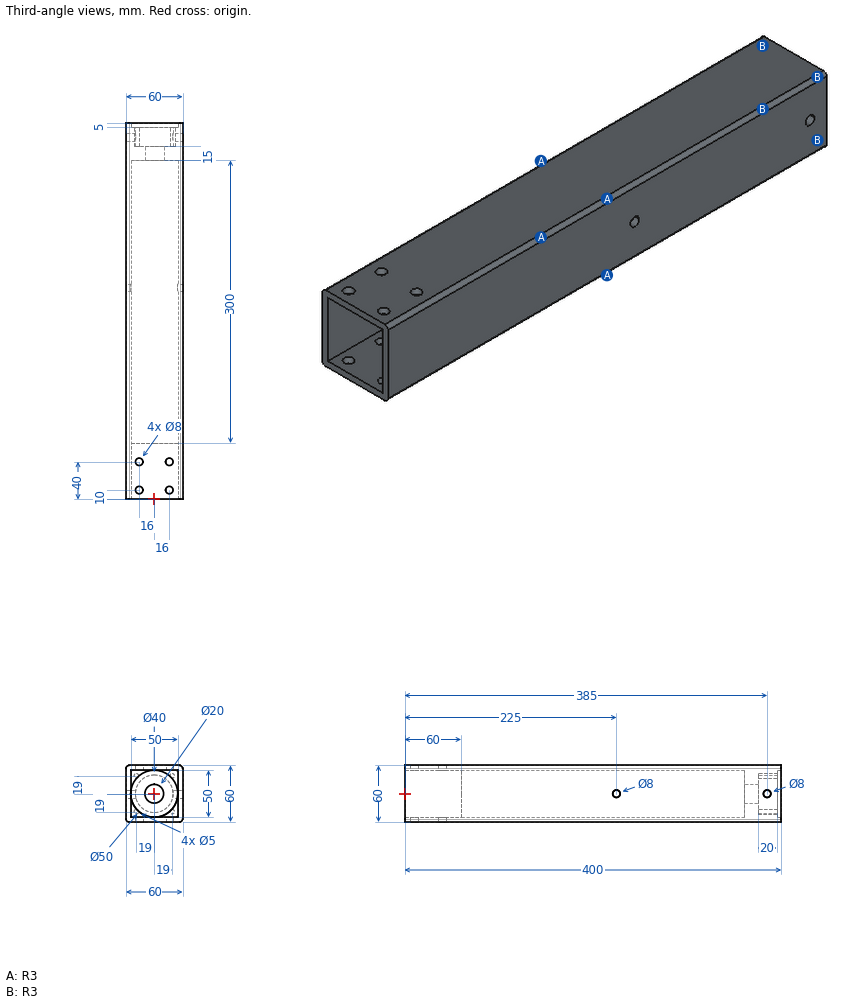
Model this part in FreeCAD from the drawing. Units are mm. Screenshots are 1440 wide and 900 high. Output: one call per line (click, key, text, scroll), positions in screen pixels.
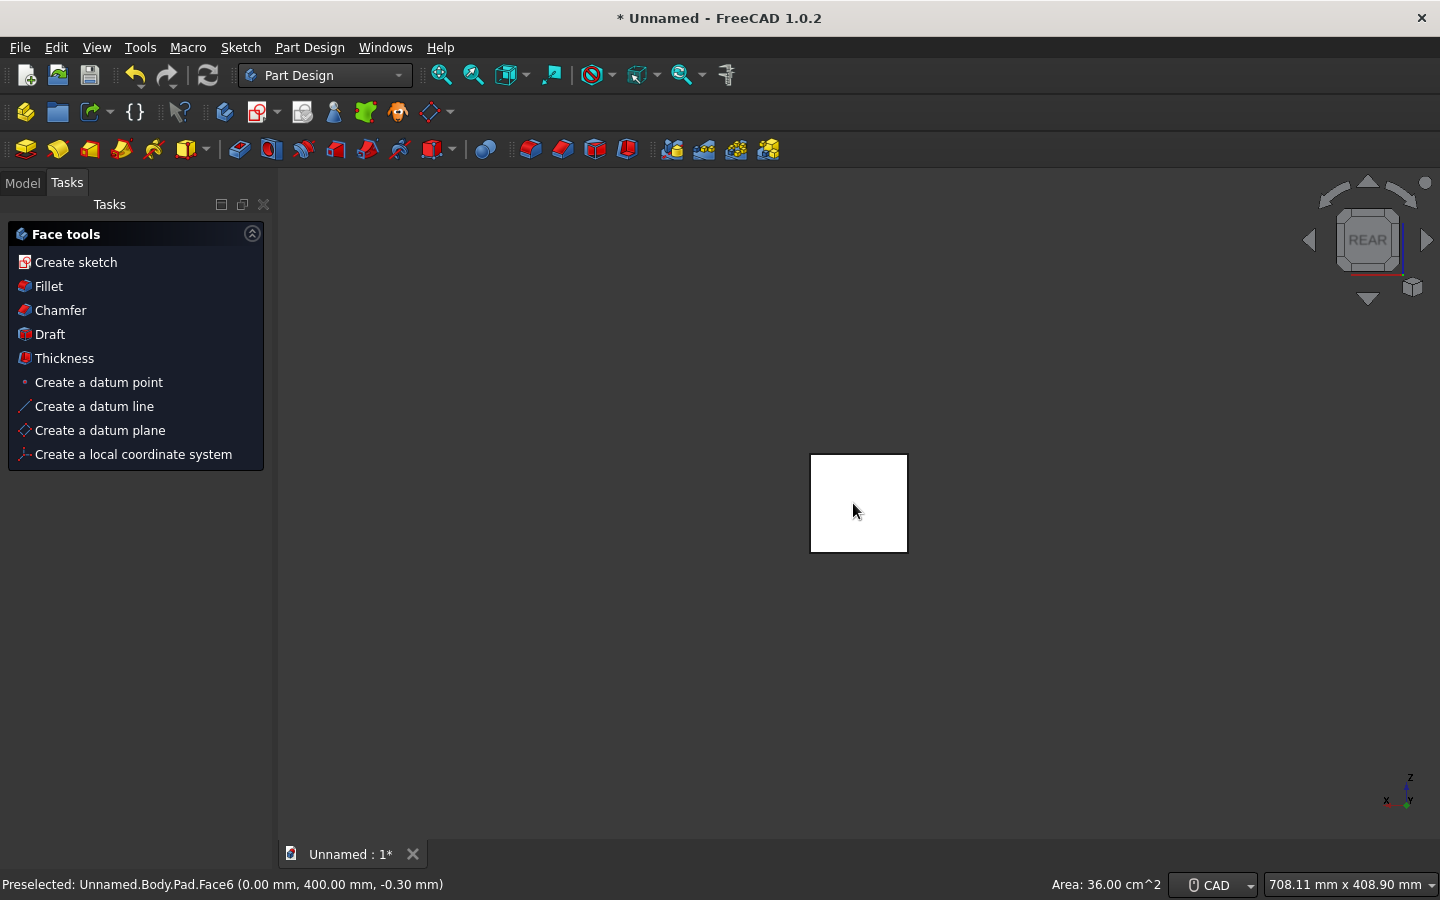
click(258, 112)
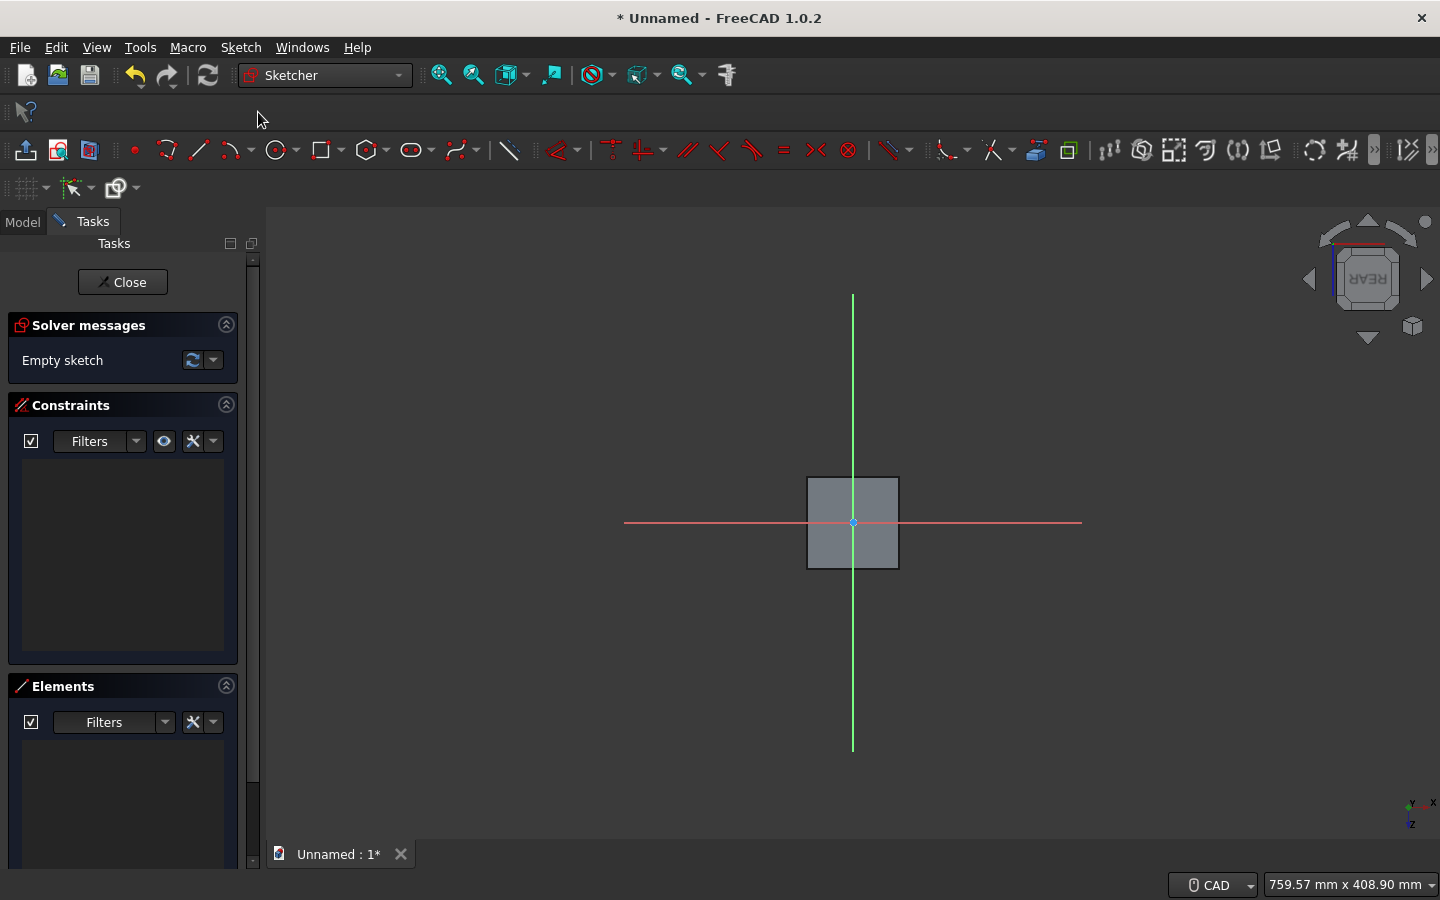
scroll(870, 523, up, 8)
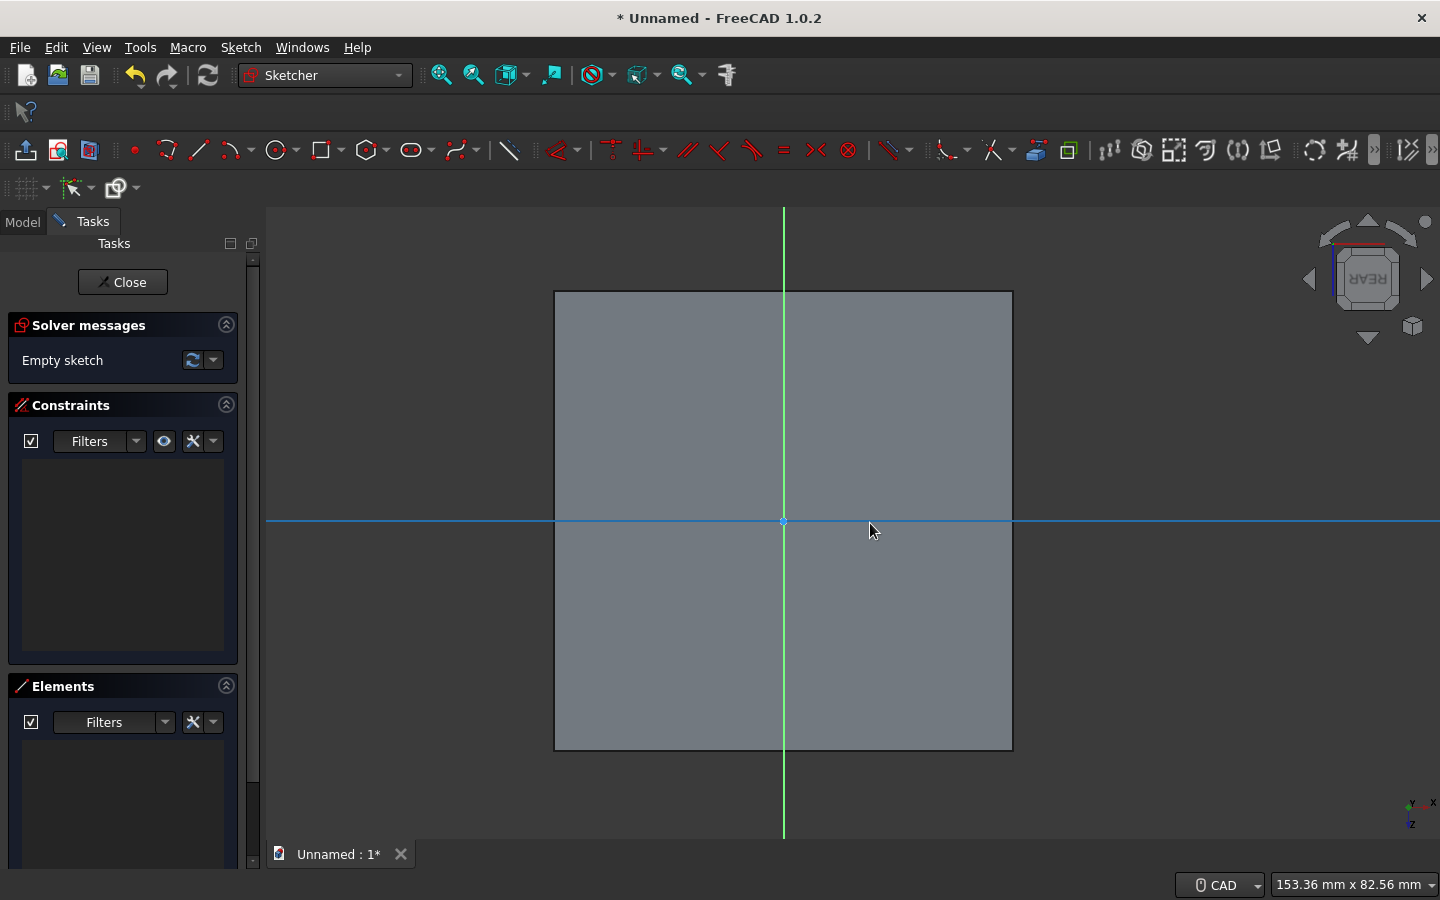
click(344, 150)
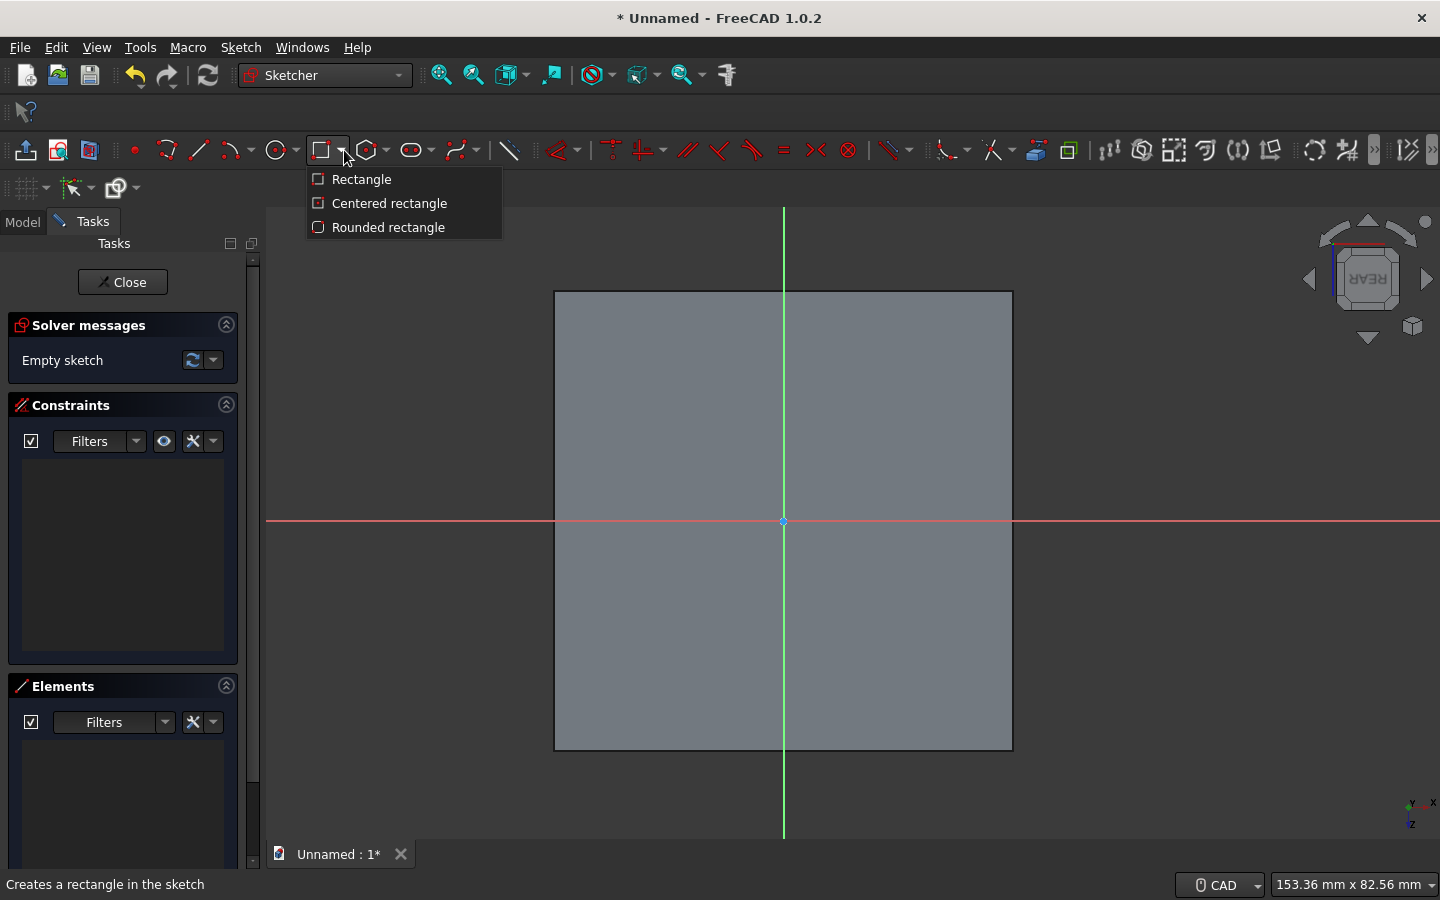
click(404, 203)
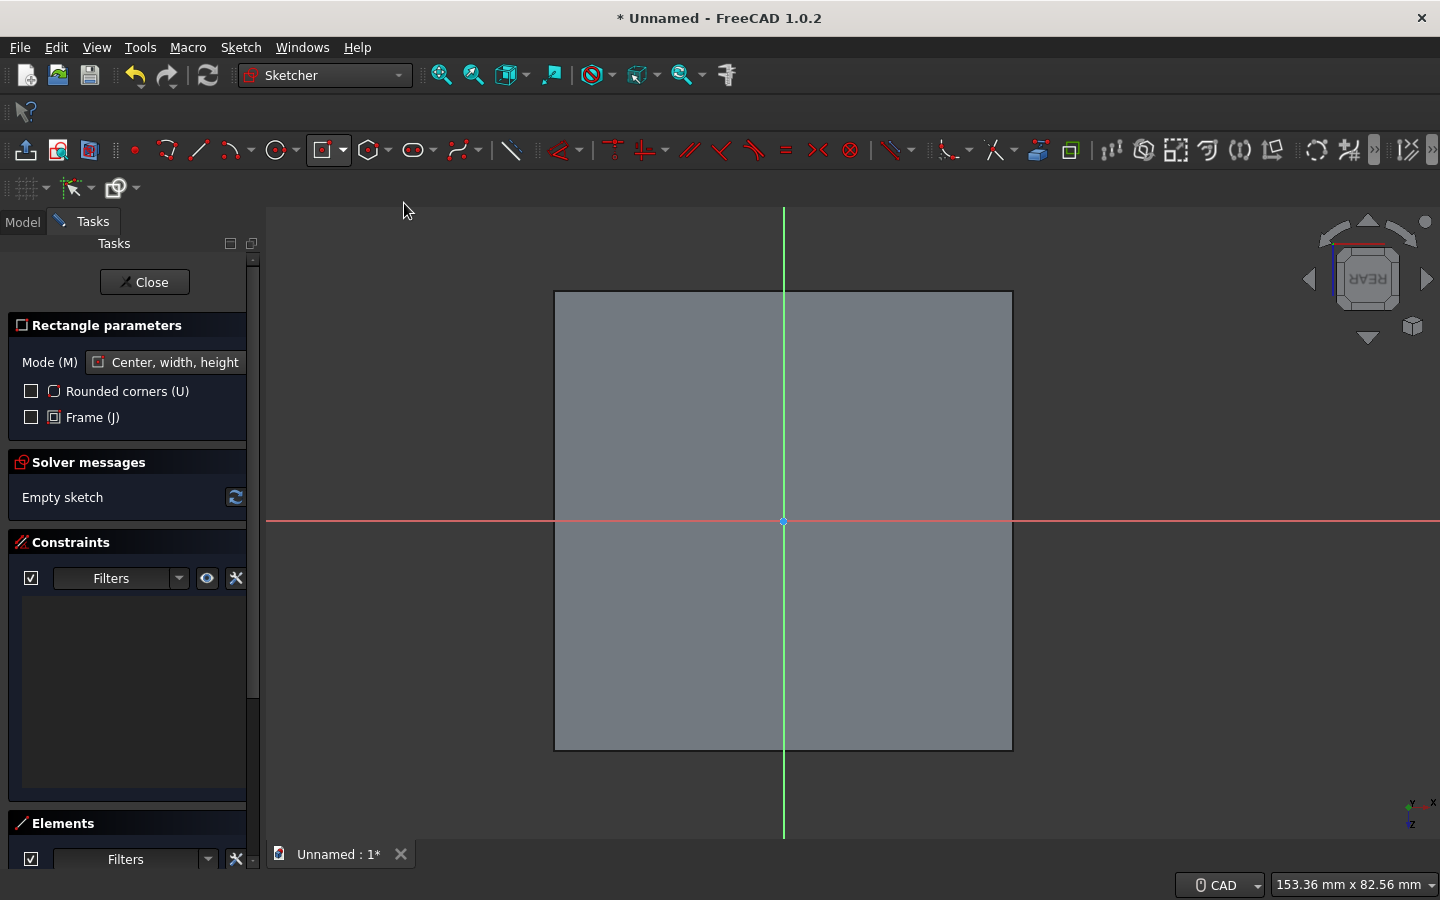
click(784, 521)
move(975, 330)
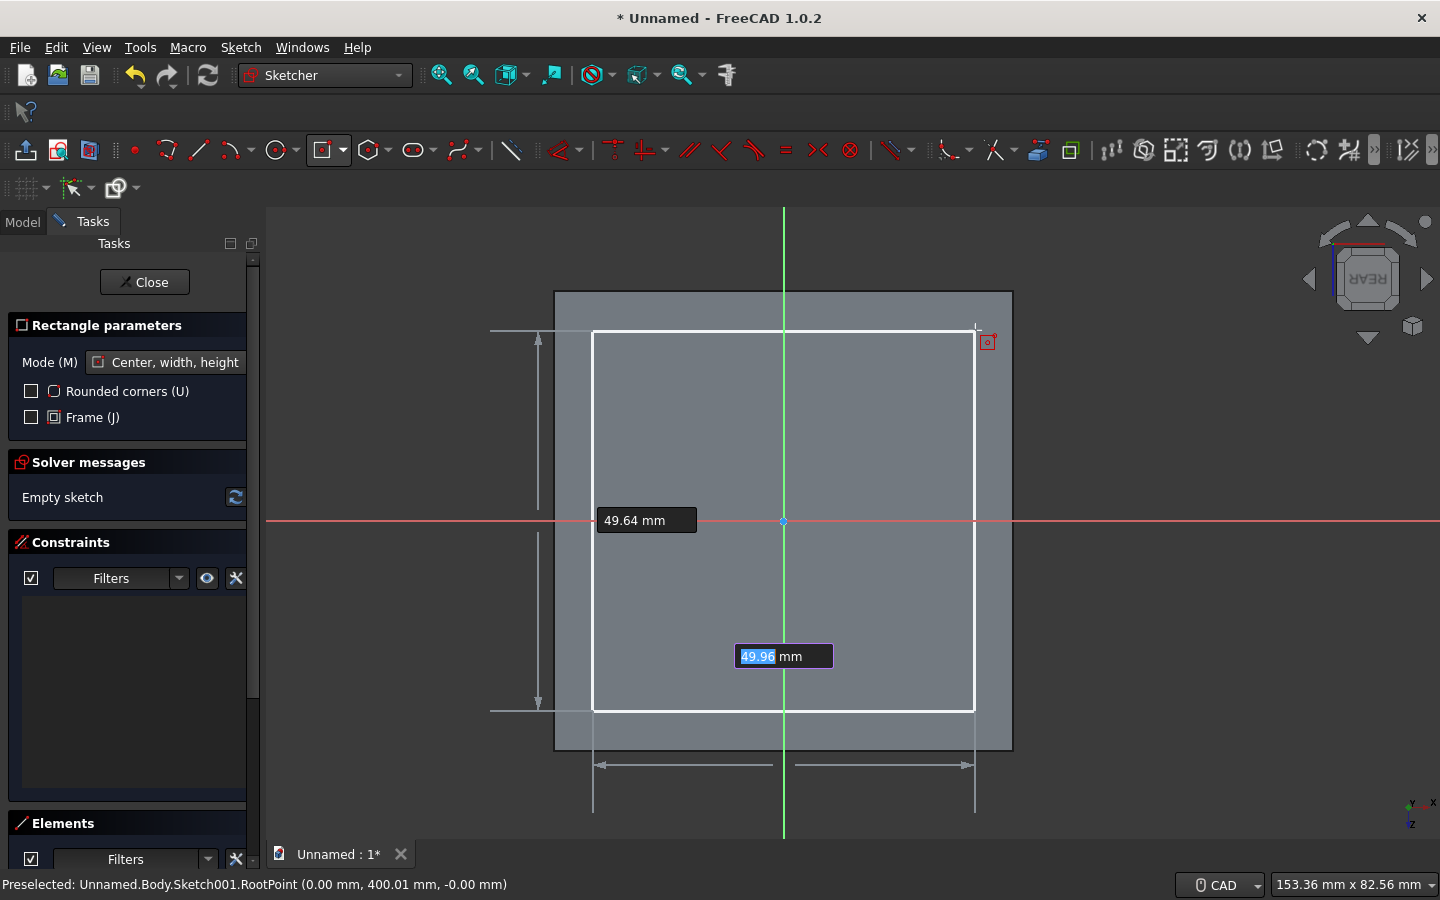
text(50)
key(Tab)
text(50)
key(Return)
key(Escape)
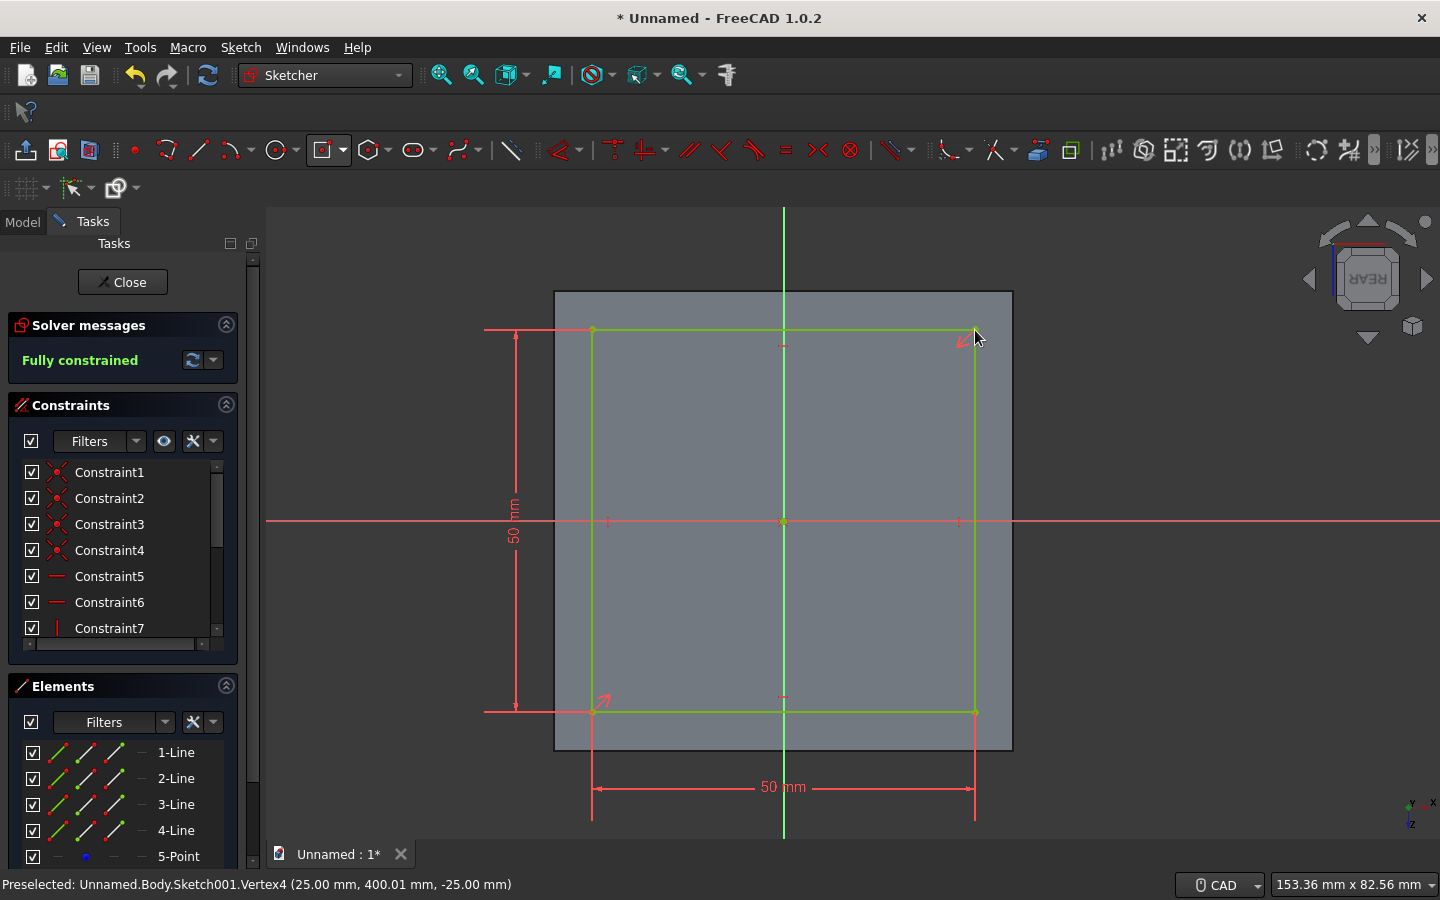
click(123, 282)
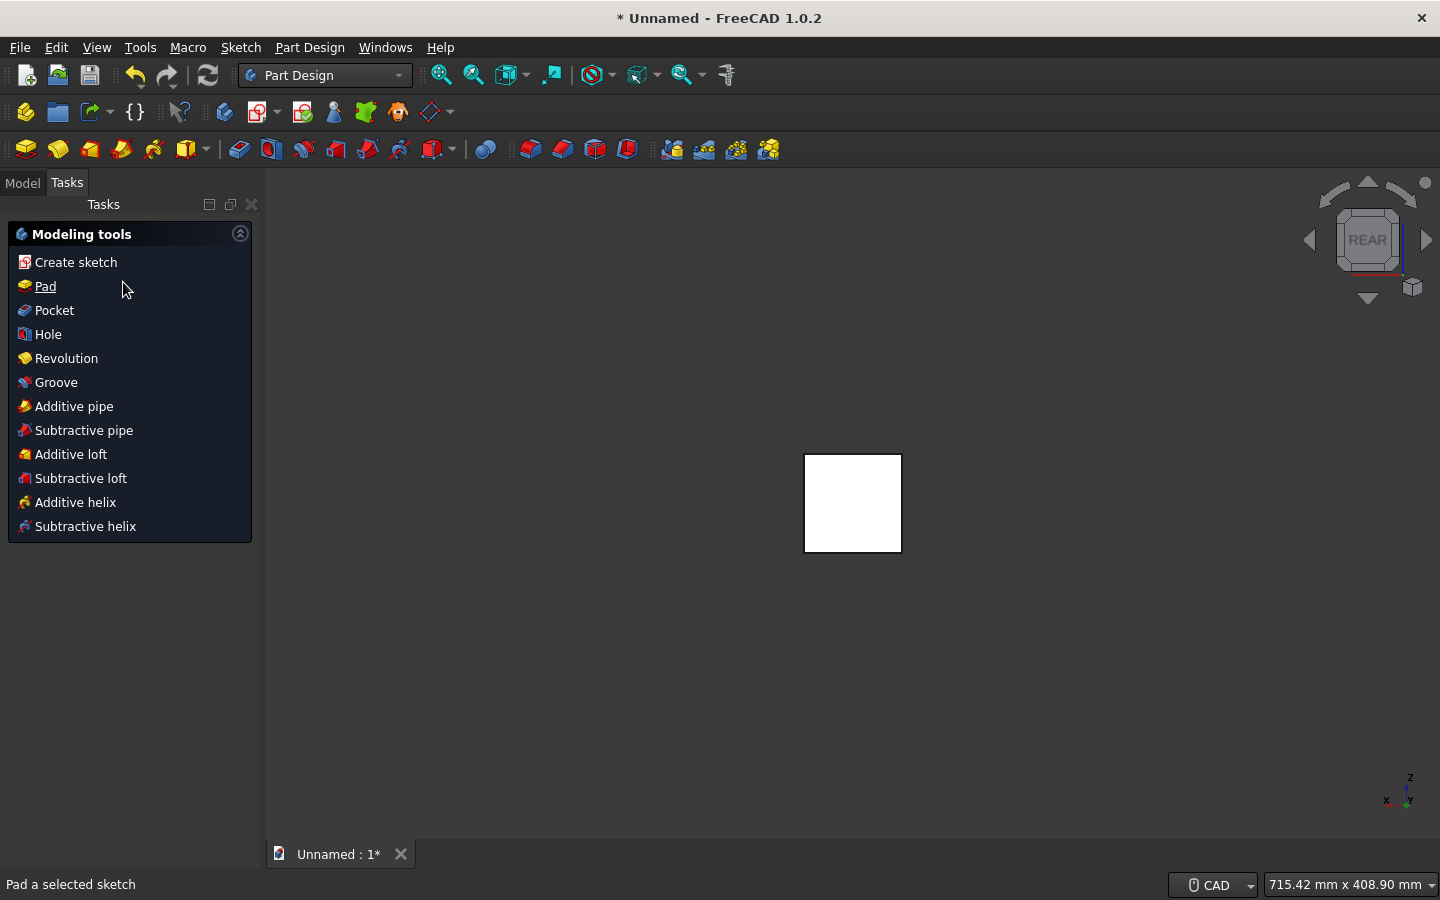
click(240, 150)